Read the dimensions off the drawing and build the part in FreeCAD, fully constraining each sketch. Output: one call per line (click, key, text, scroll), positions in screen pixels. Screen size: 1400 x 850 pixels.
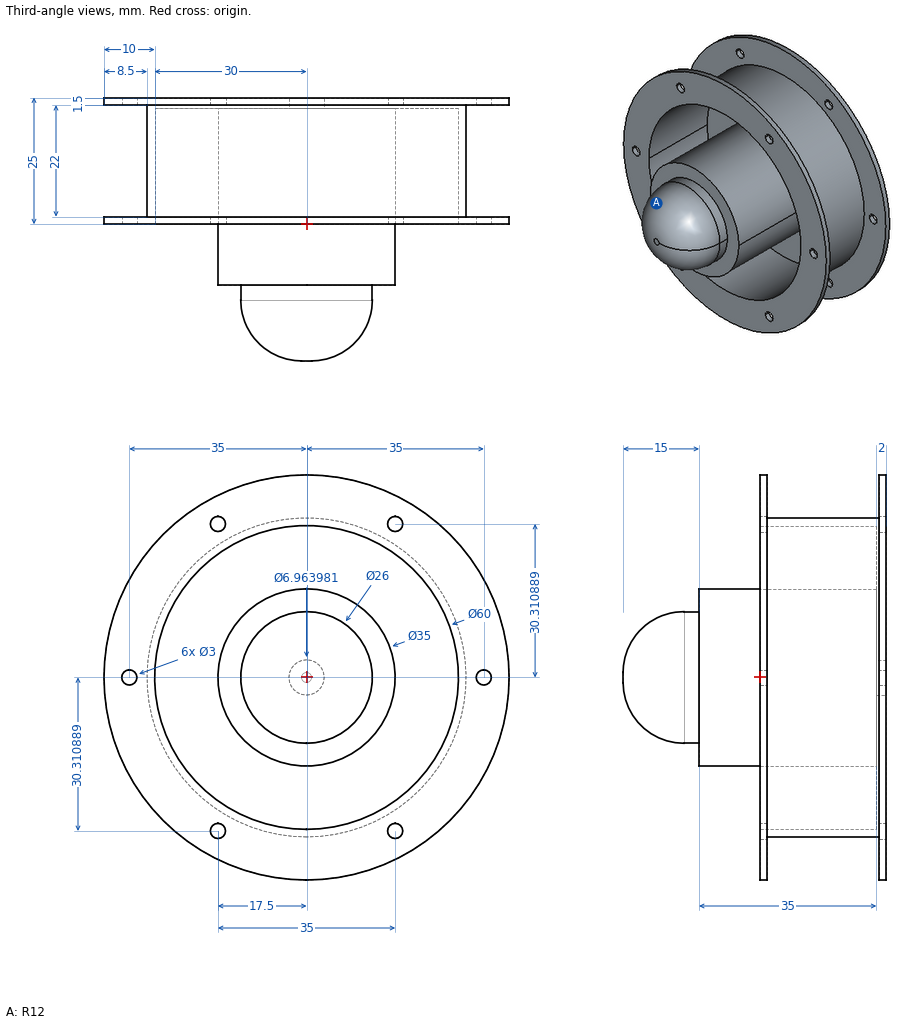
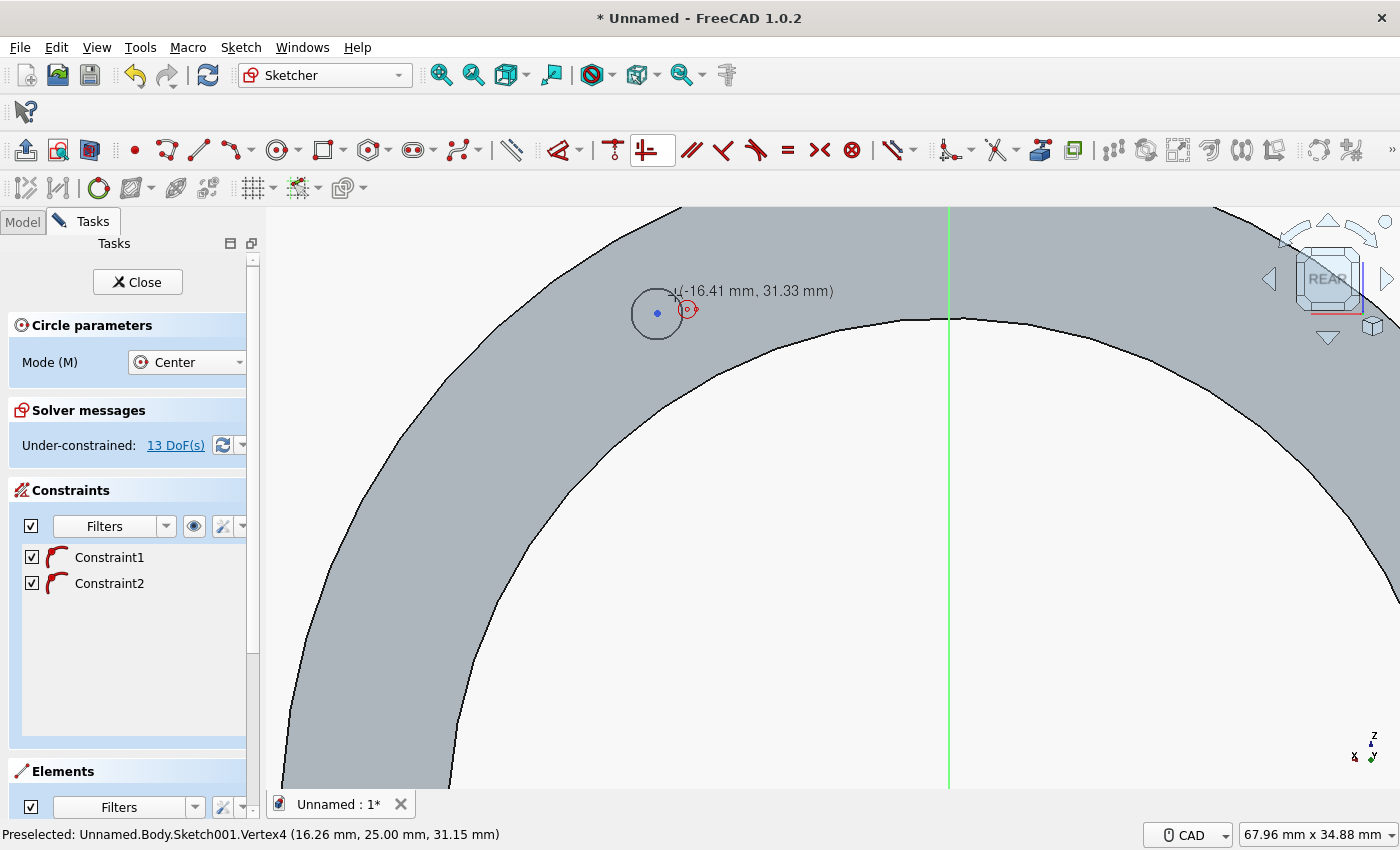
scroll(657, 311, down, 5)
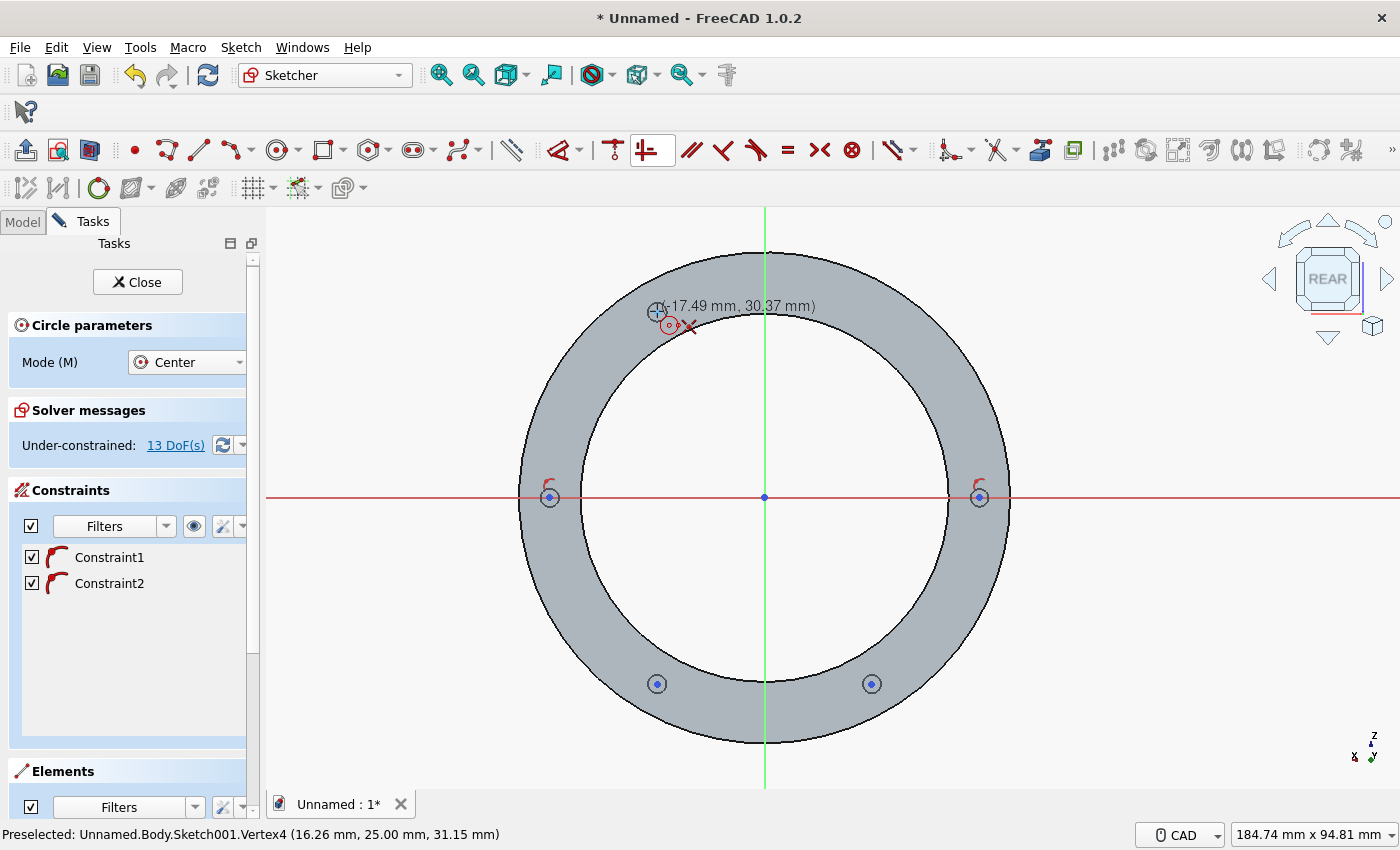
scroll(872, 312, up, 5)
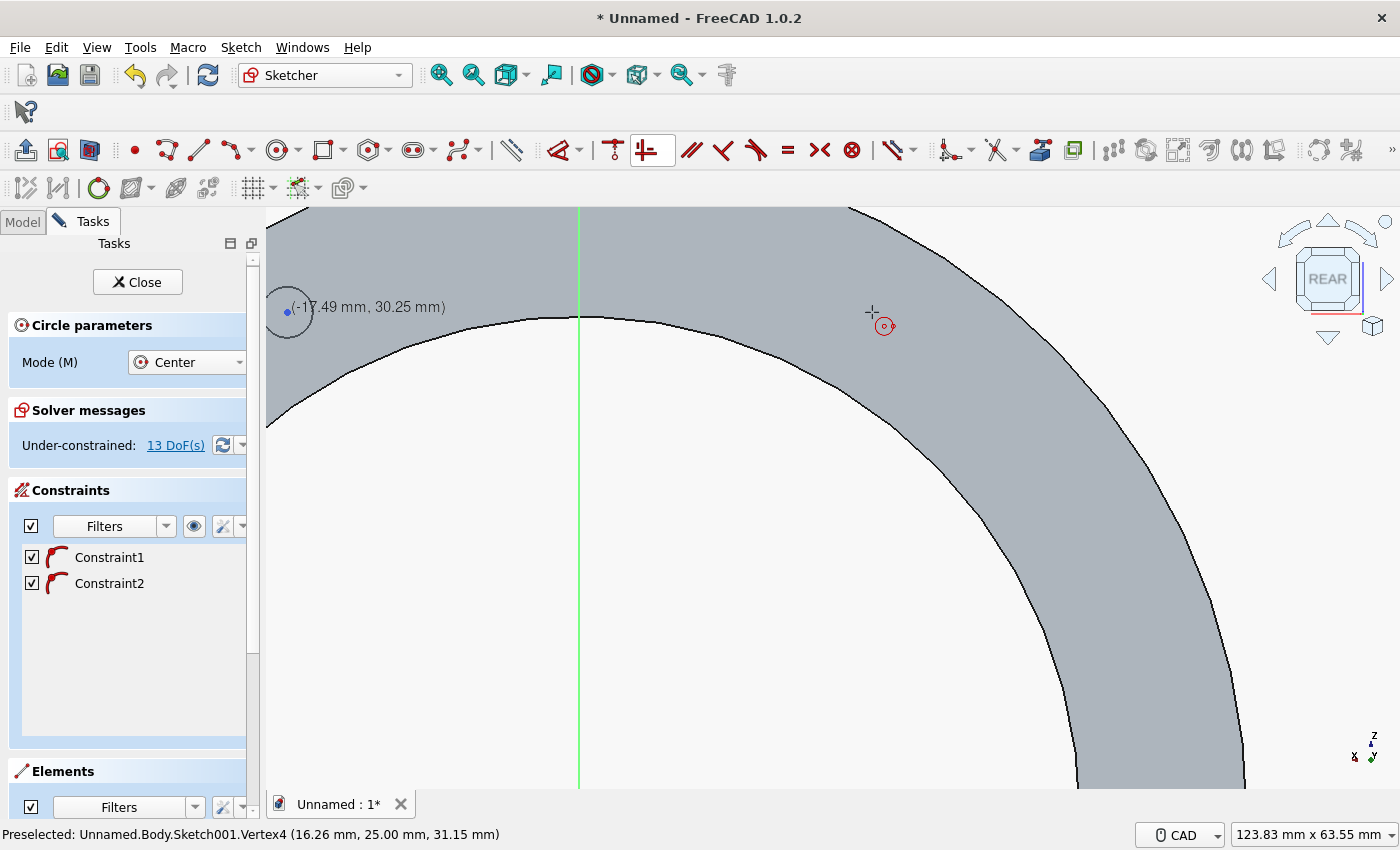
click(871, 311)
click(889, 294)
key(Escape)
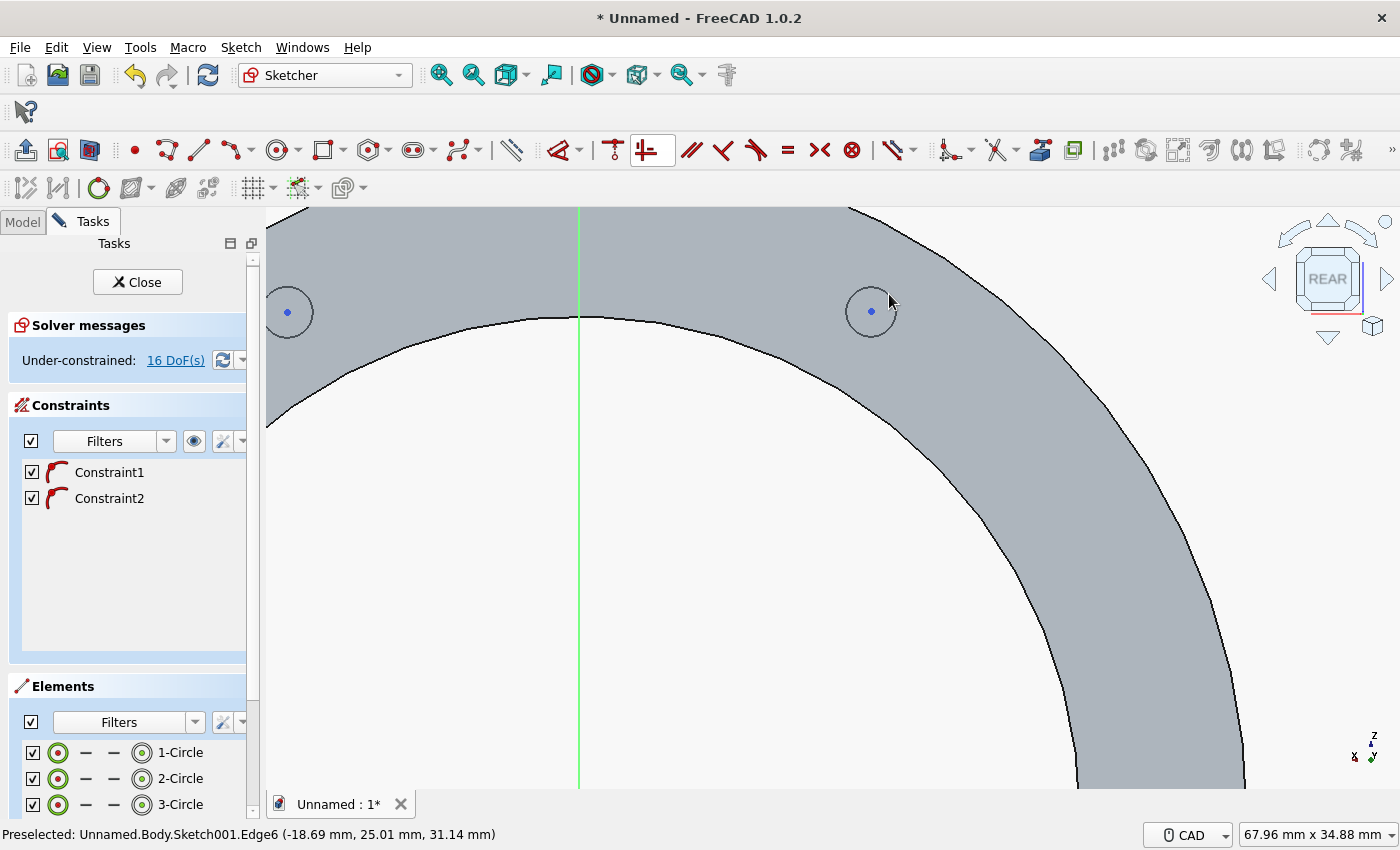
scroll(872, 312, down, 5)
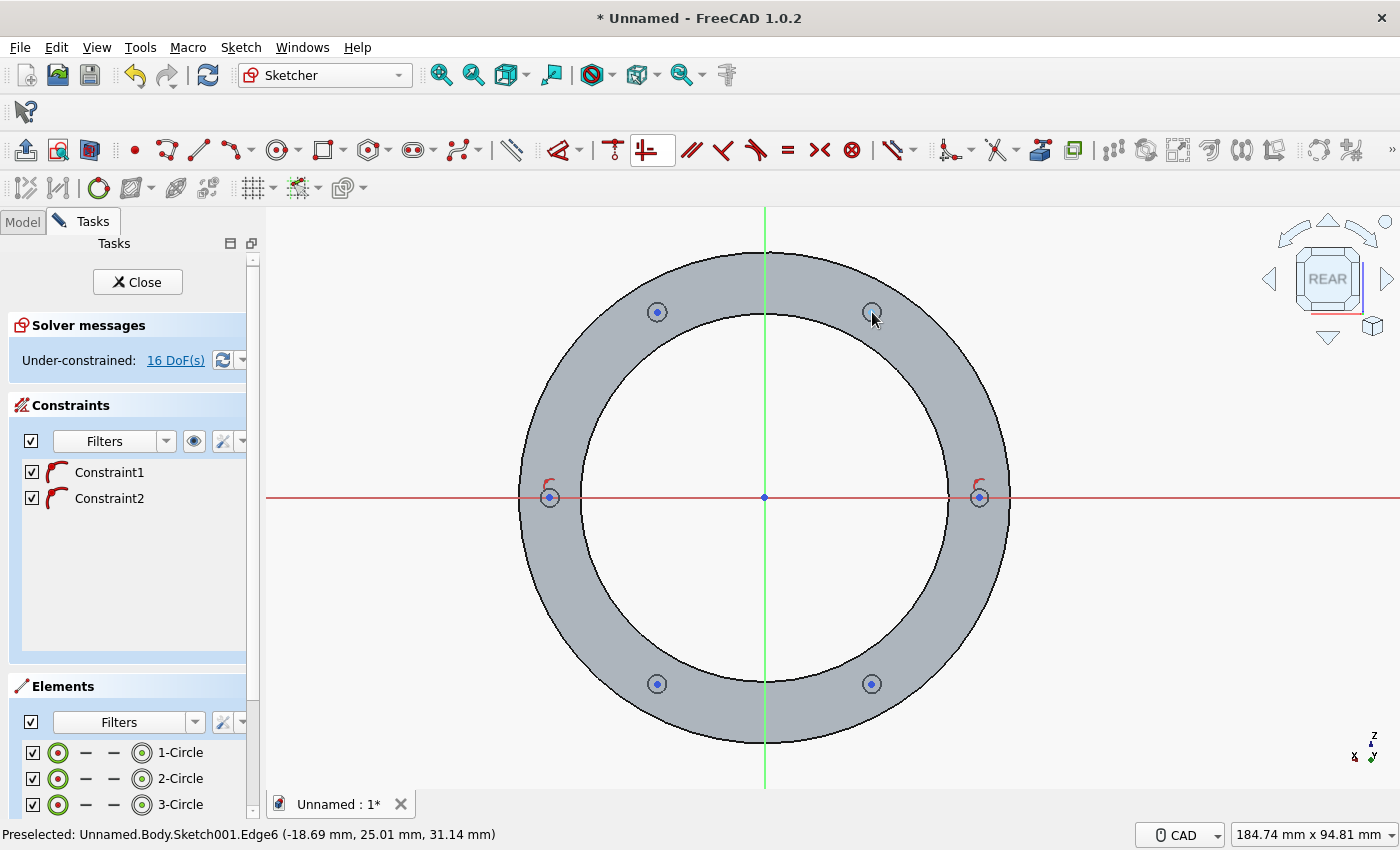
scroll(986, 492, up, 4)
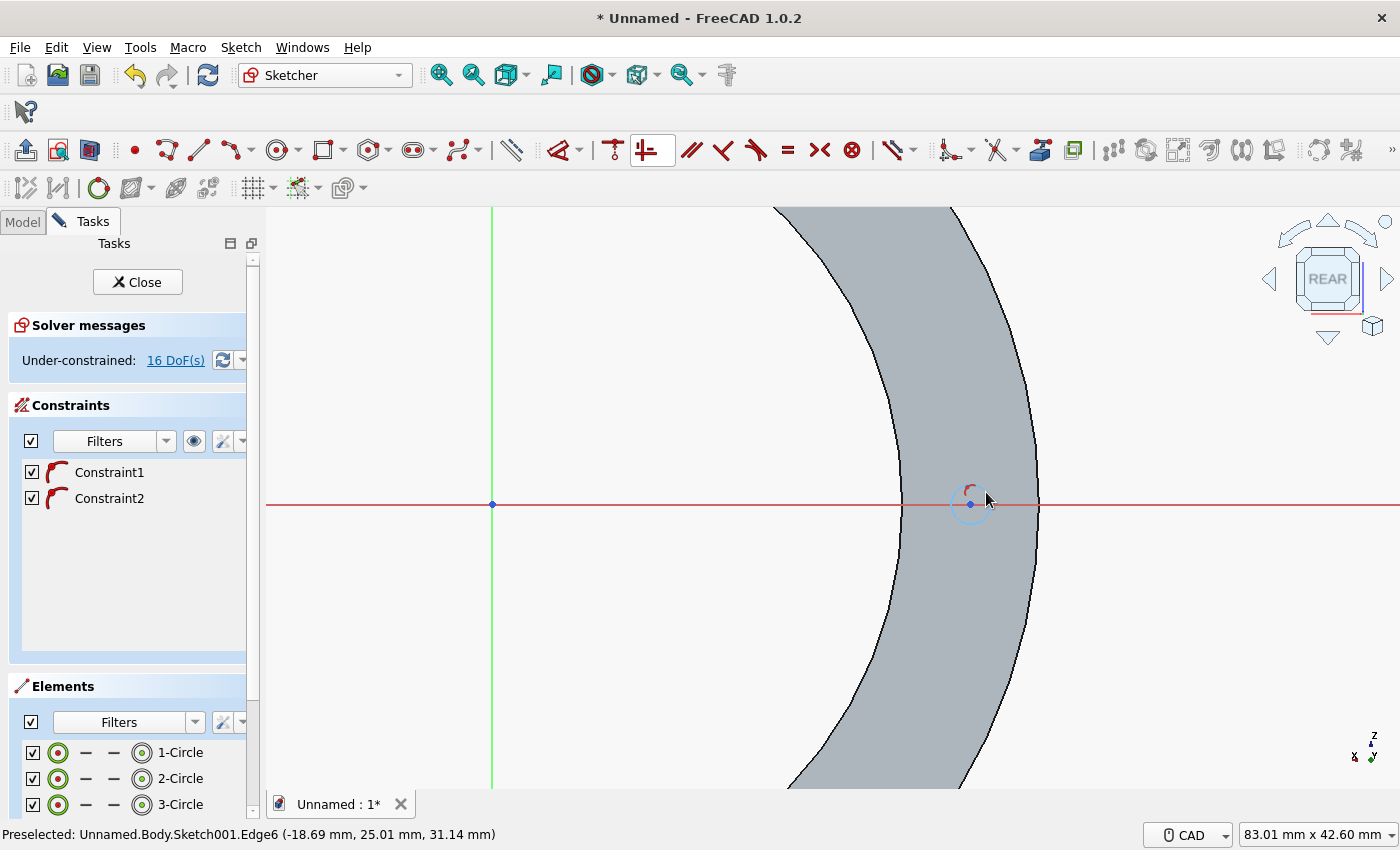
click(985, 491)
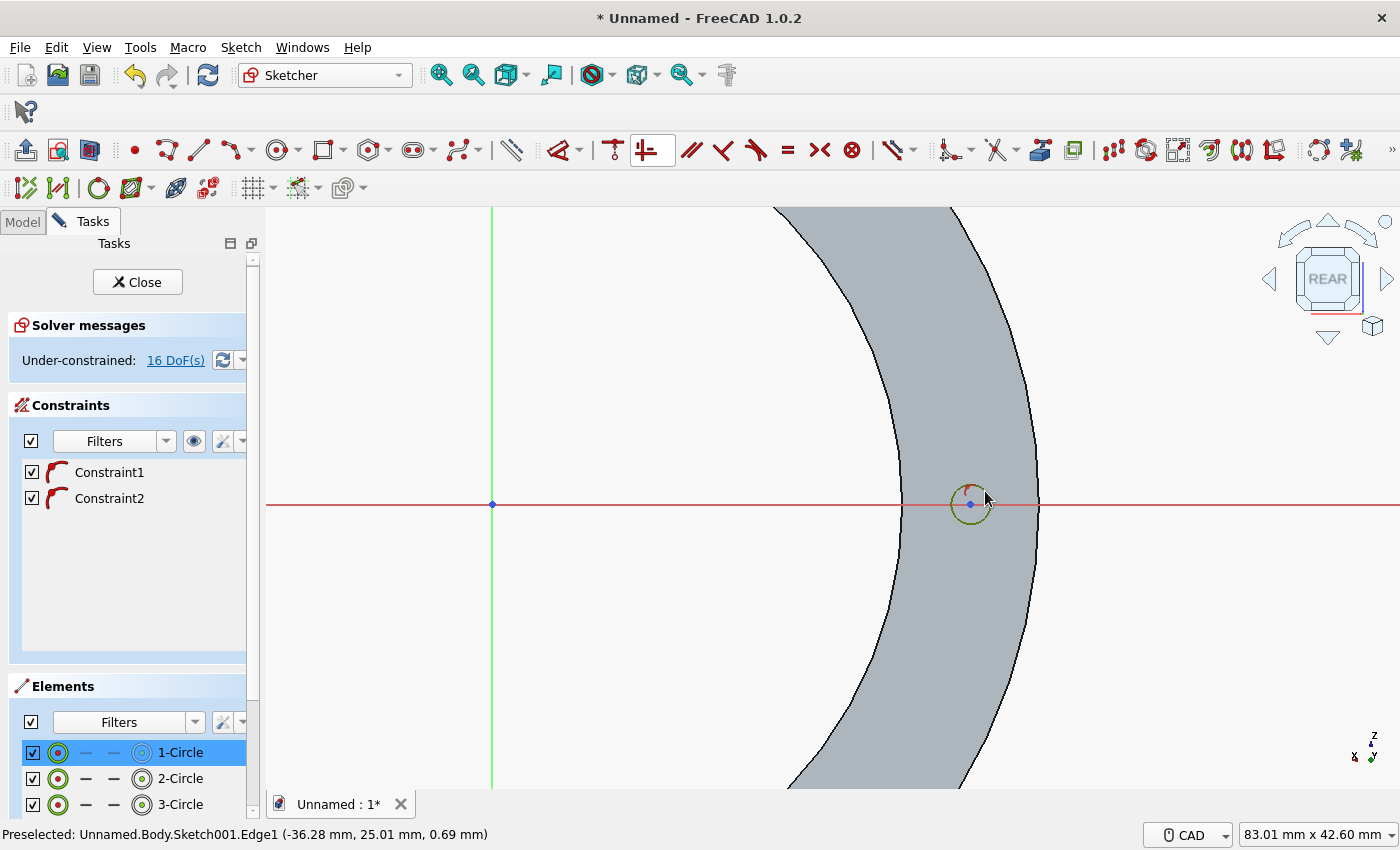
scroll(986, 493, down, 4)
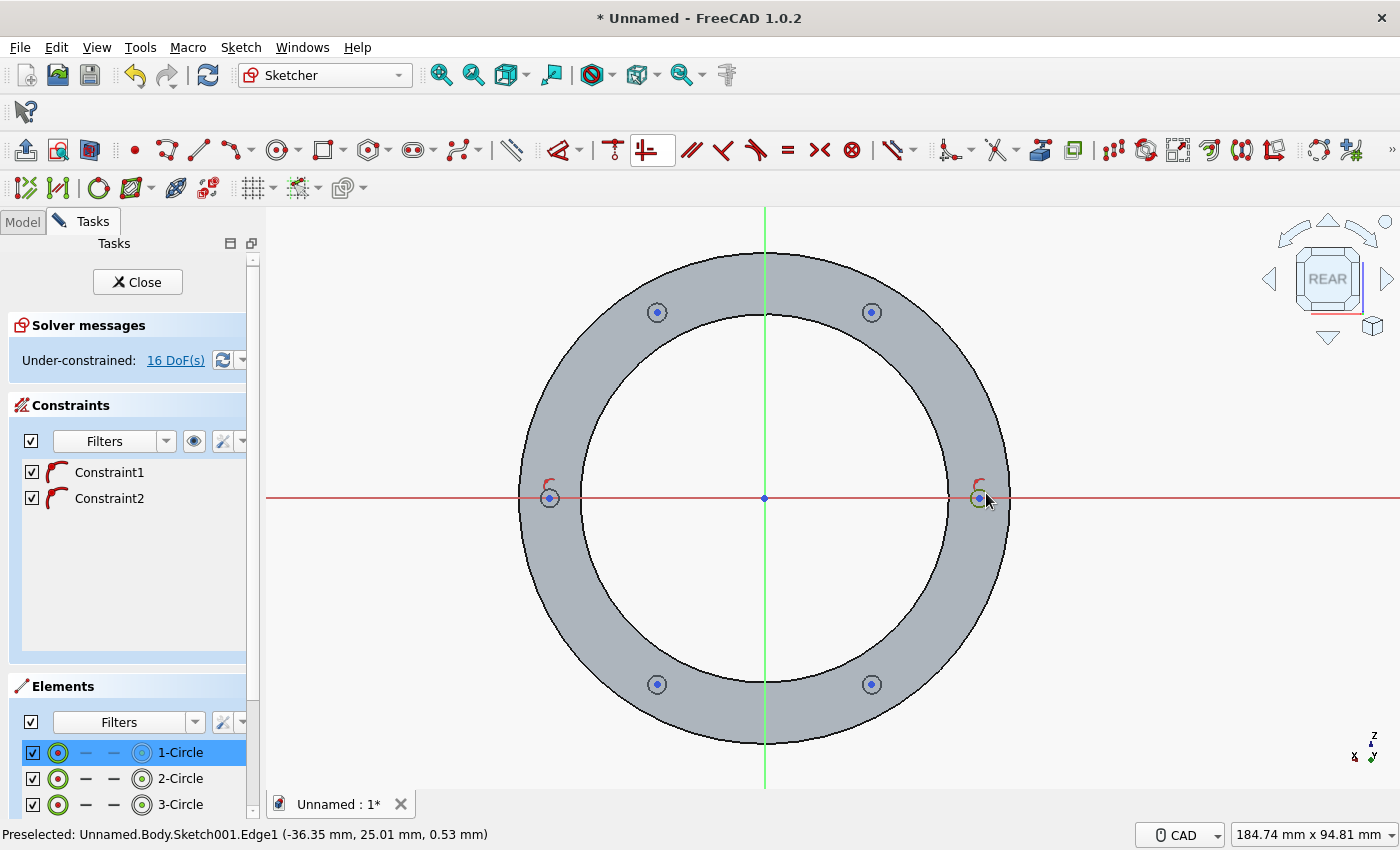
scroll(878, 678, up, 3)